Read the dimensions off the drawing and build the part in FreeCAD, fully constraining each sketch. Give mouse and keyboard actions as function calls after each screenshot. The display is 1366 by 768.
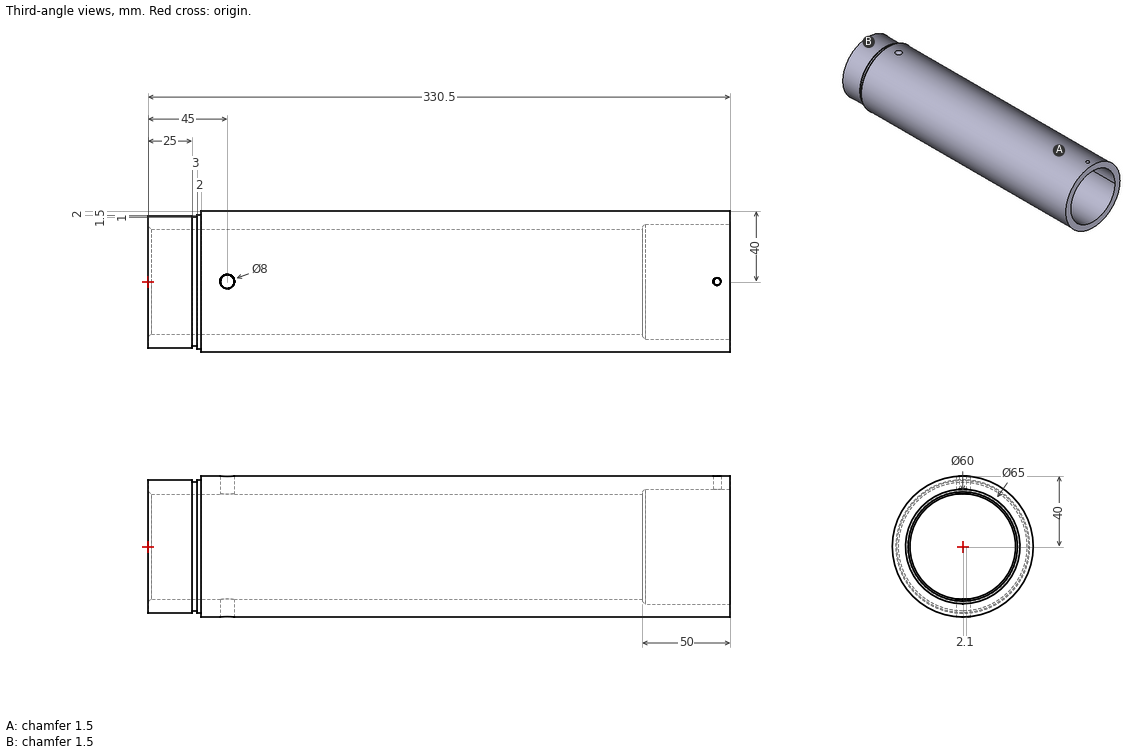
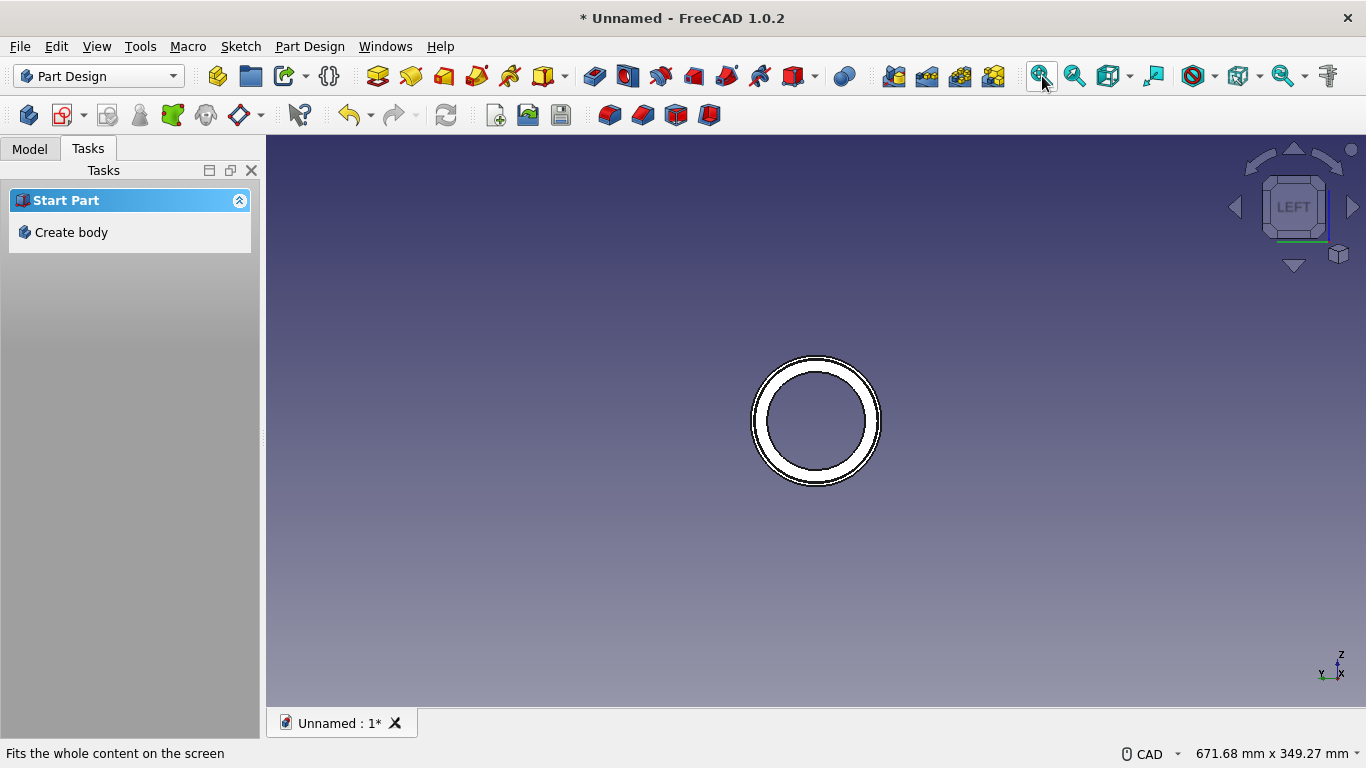
key(v)
key(3)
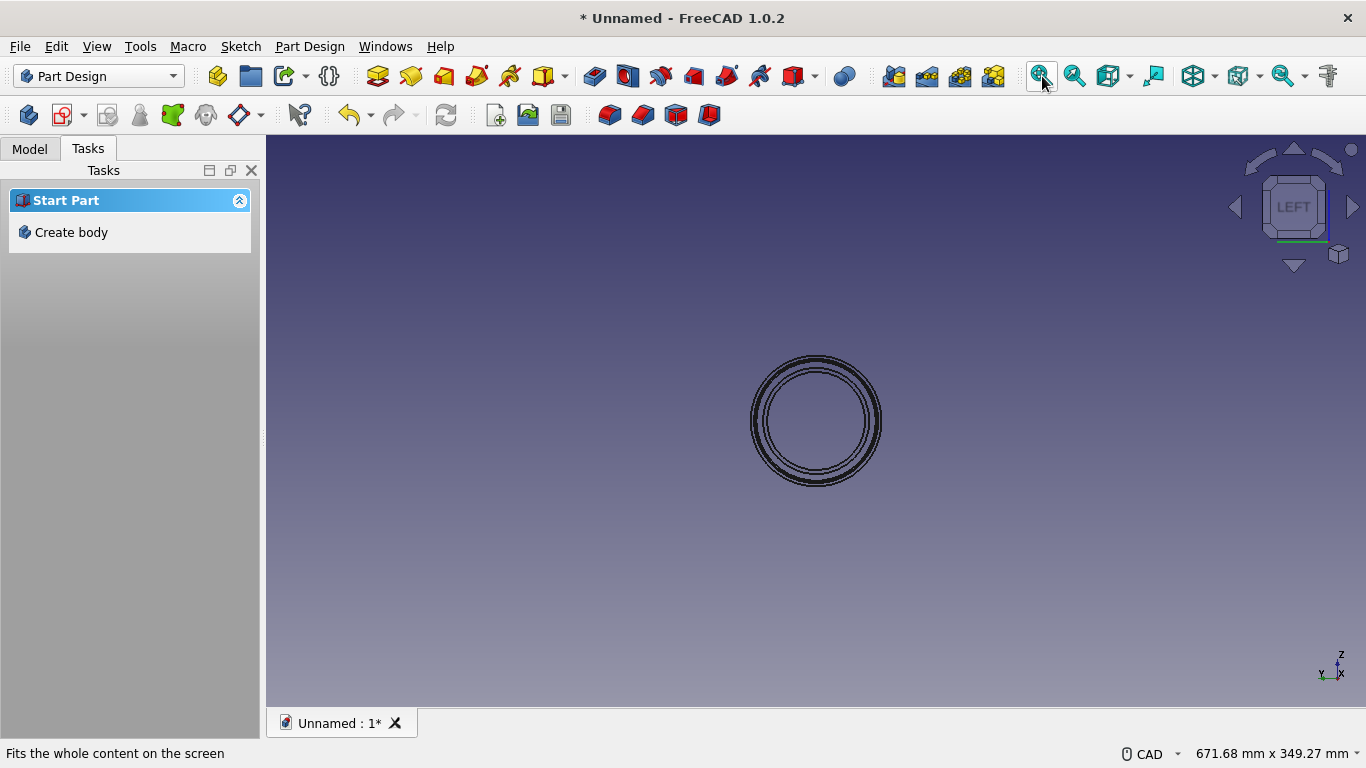
key(0)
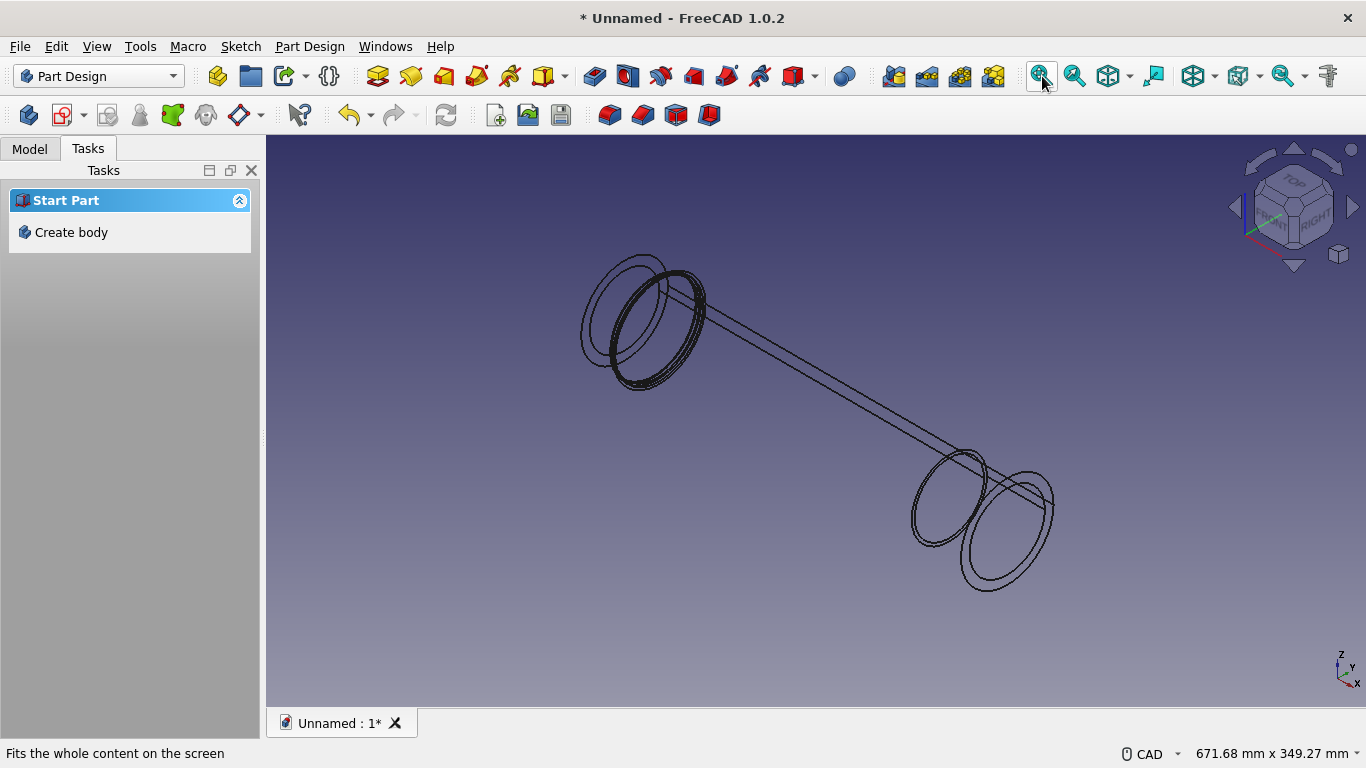
click(912, 519)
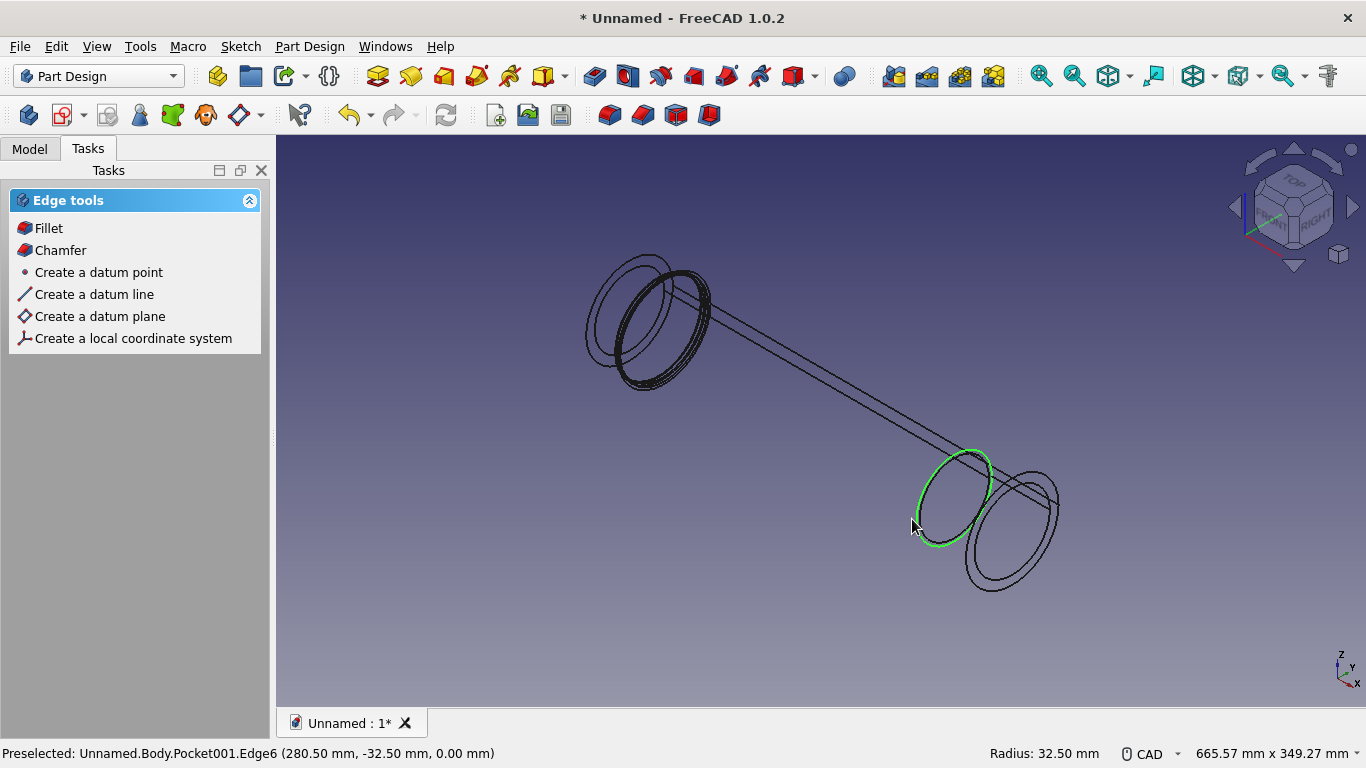
key(v)
key(1)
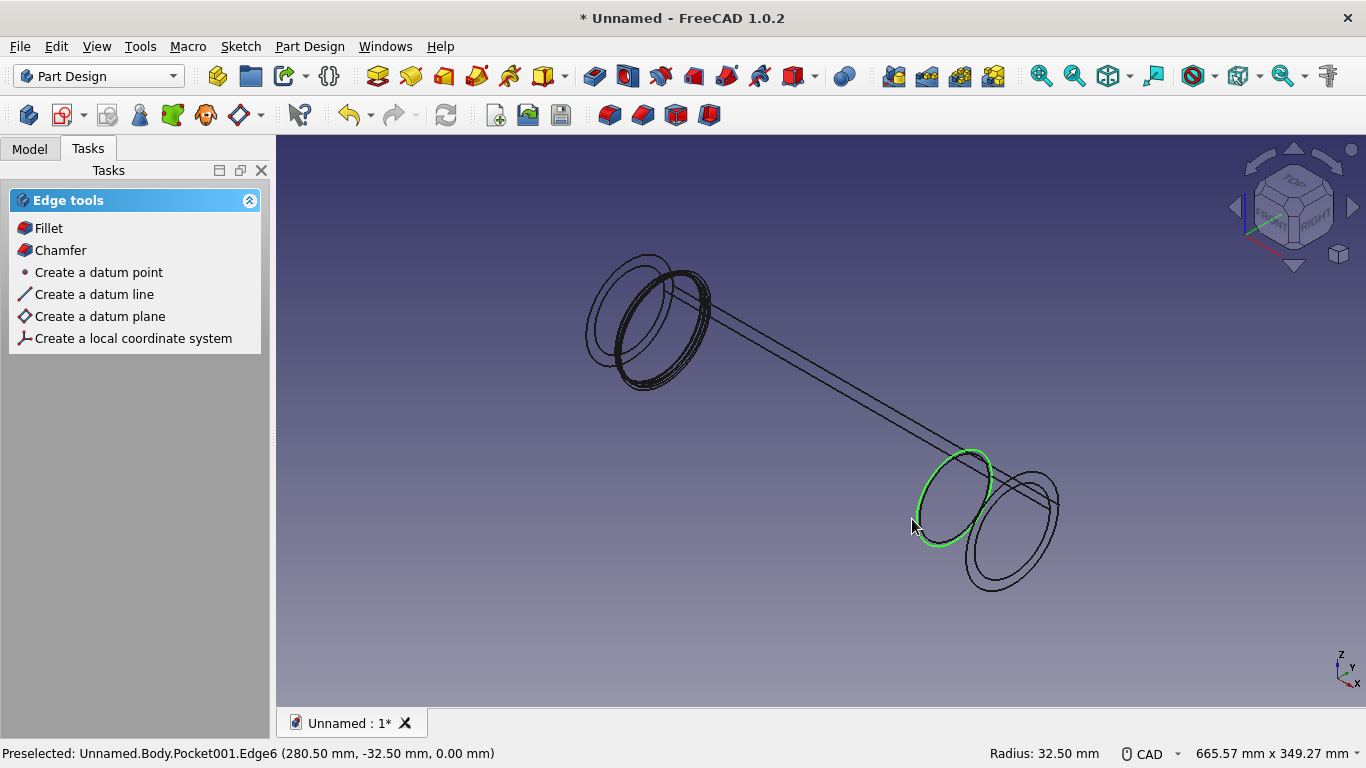
click(643, 116)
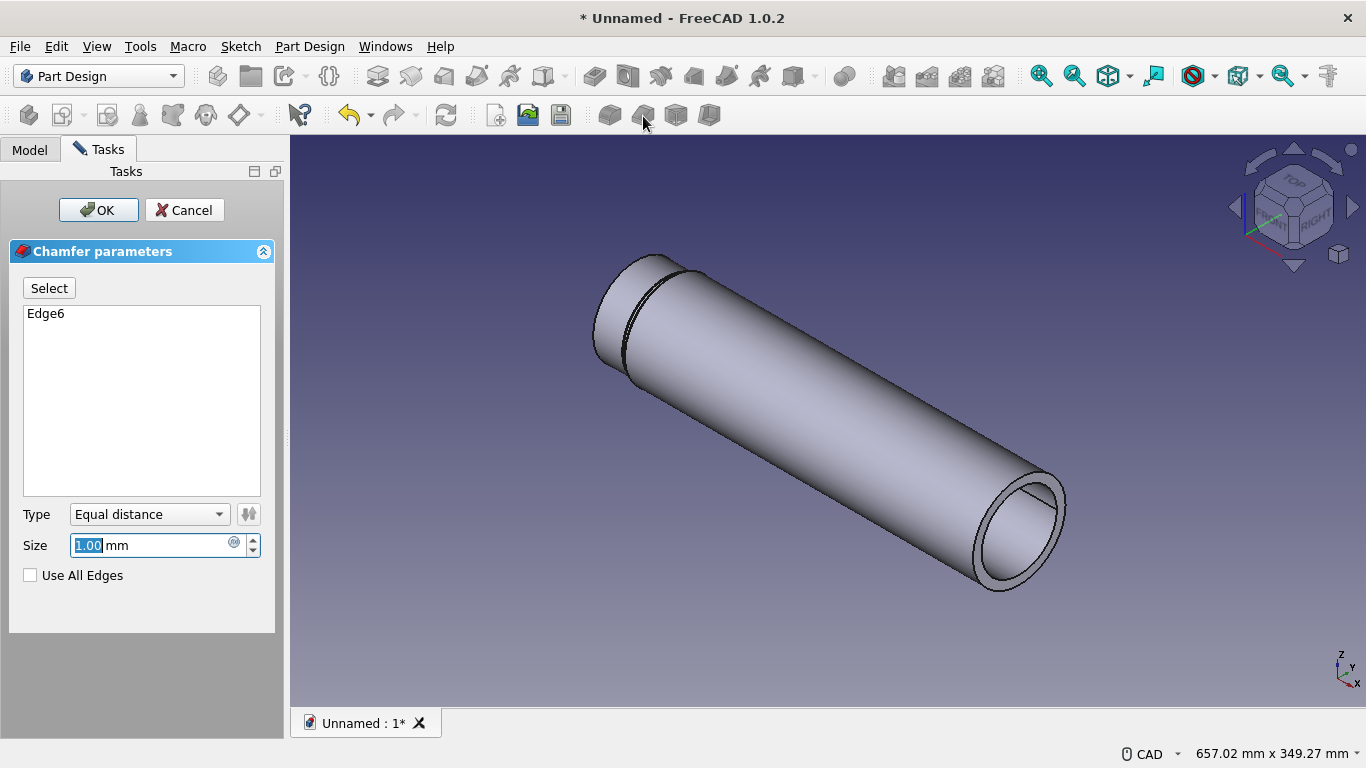
text(1.5)
key(Tab)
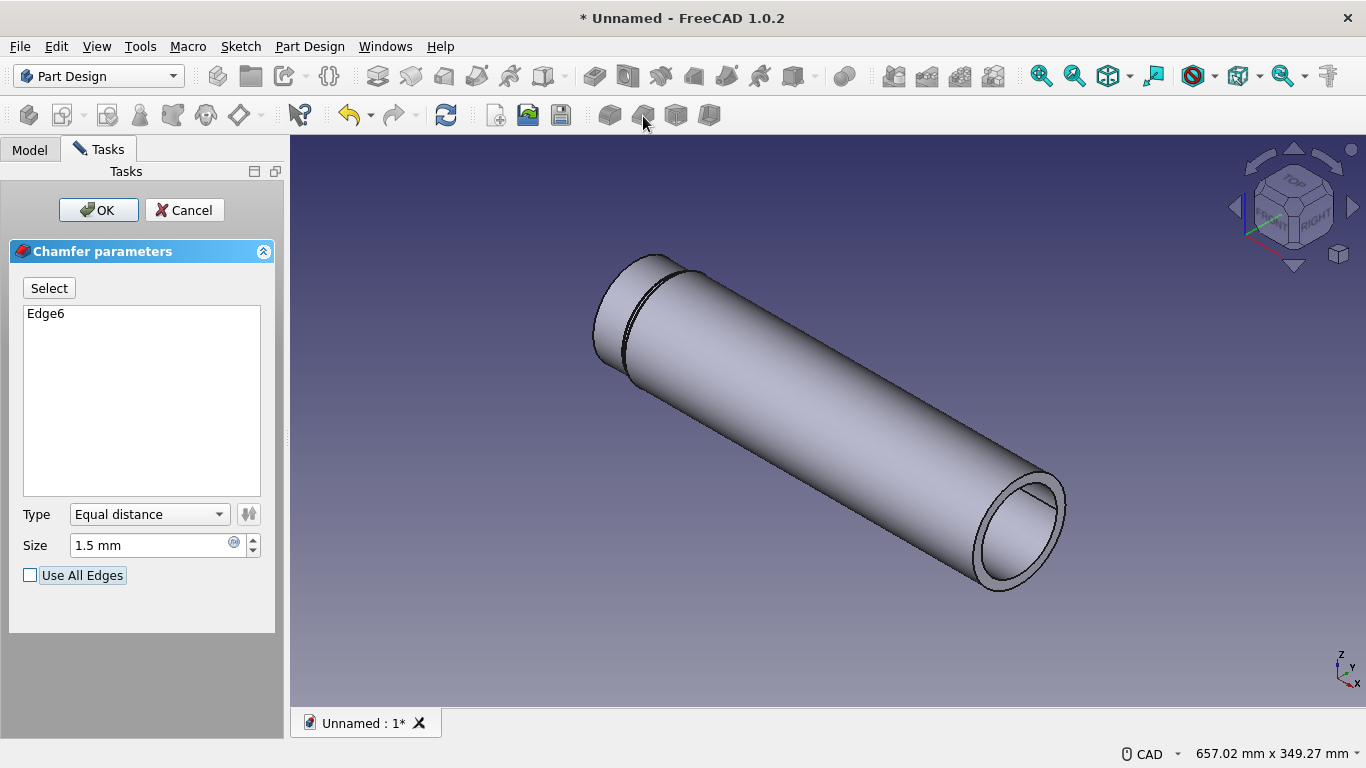
click(99, 210)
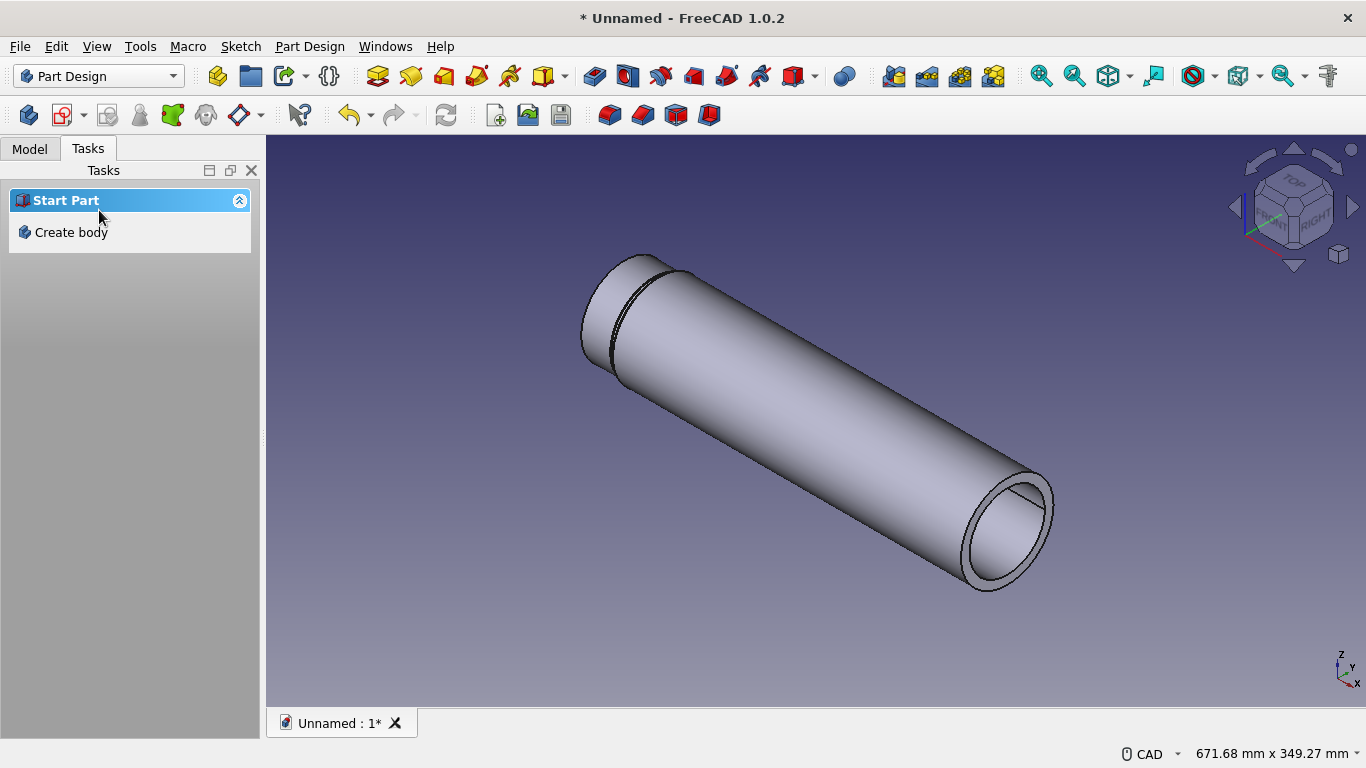
key(2)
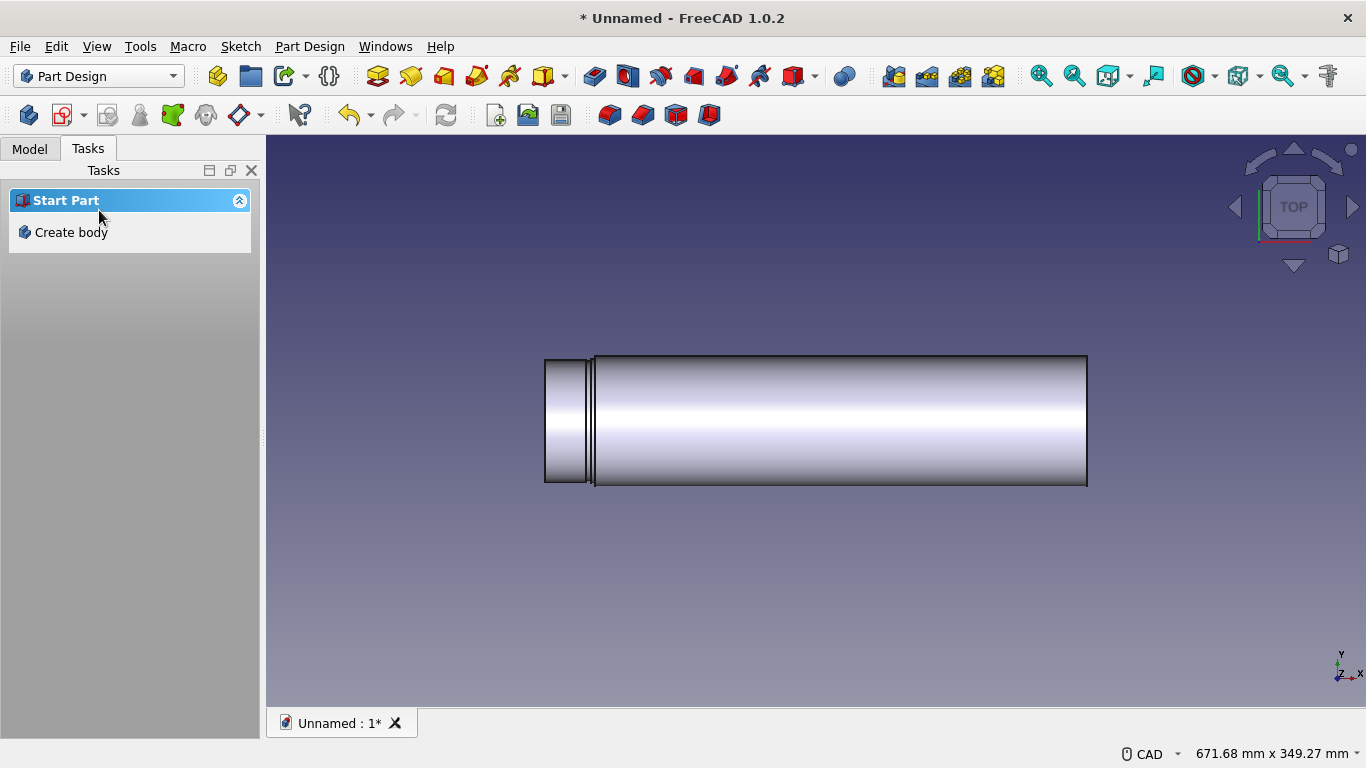
key(0)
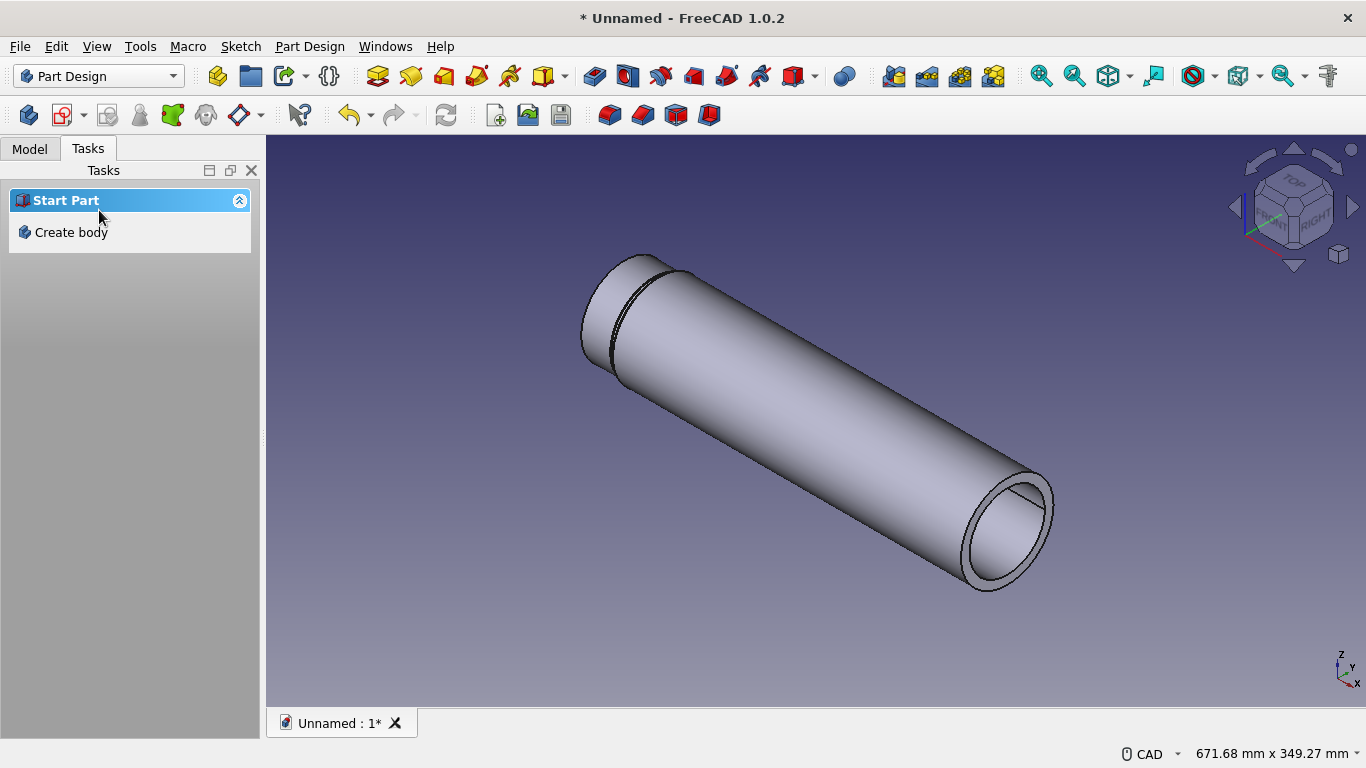
key(1)